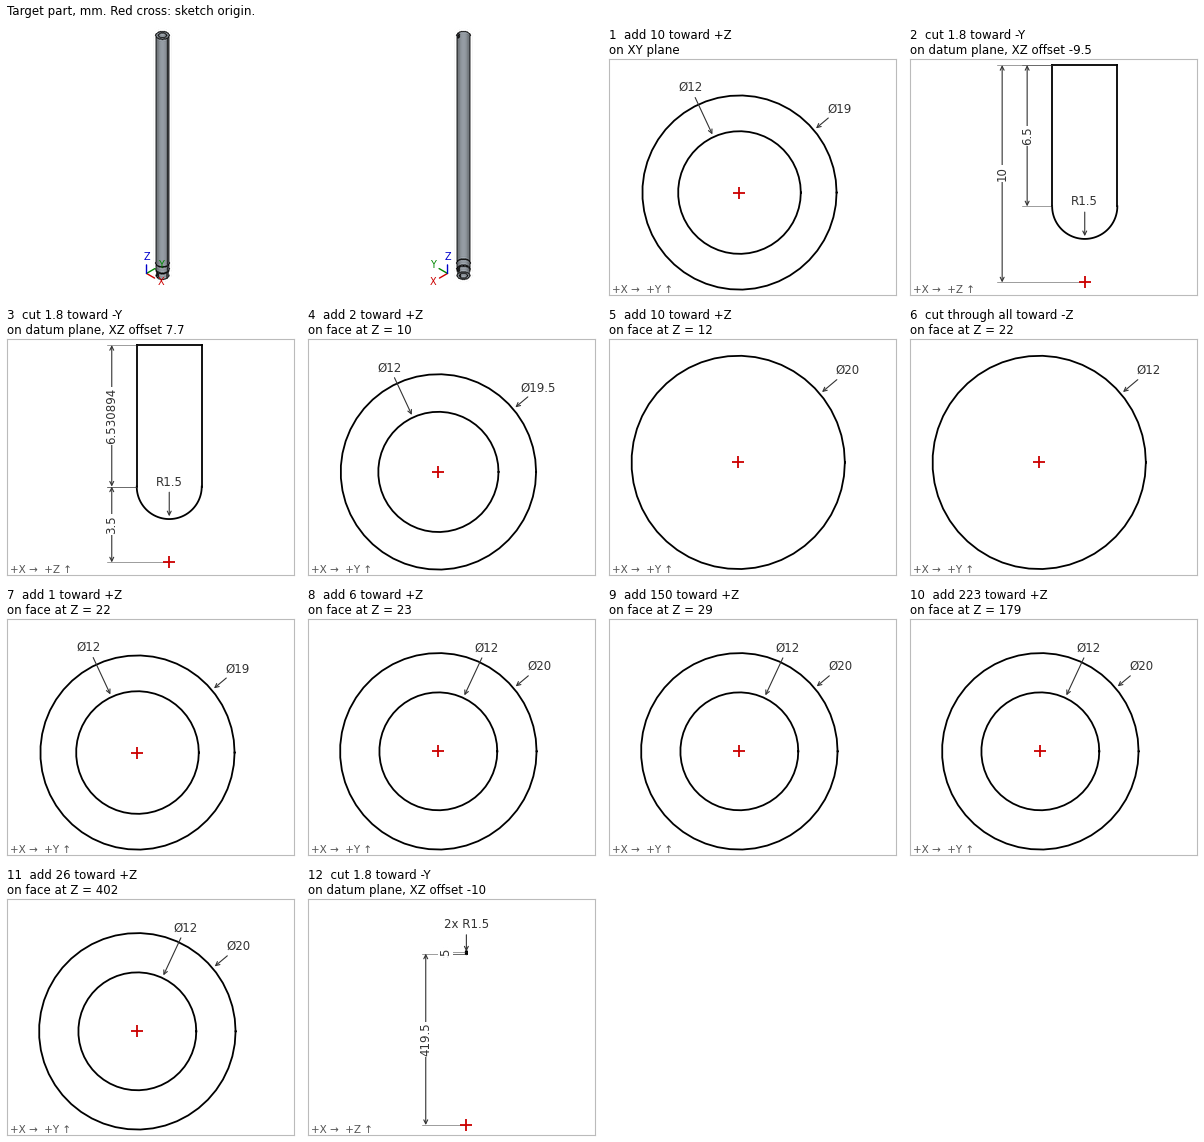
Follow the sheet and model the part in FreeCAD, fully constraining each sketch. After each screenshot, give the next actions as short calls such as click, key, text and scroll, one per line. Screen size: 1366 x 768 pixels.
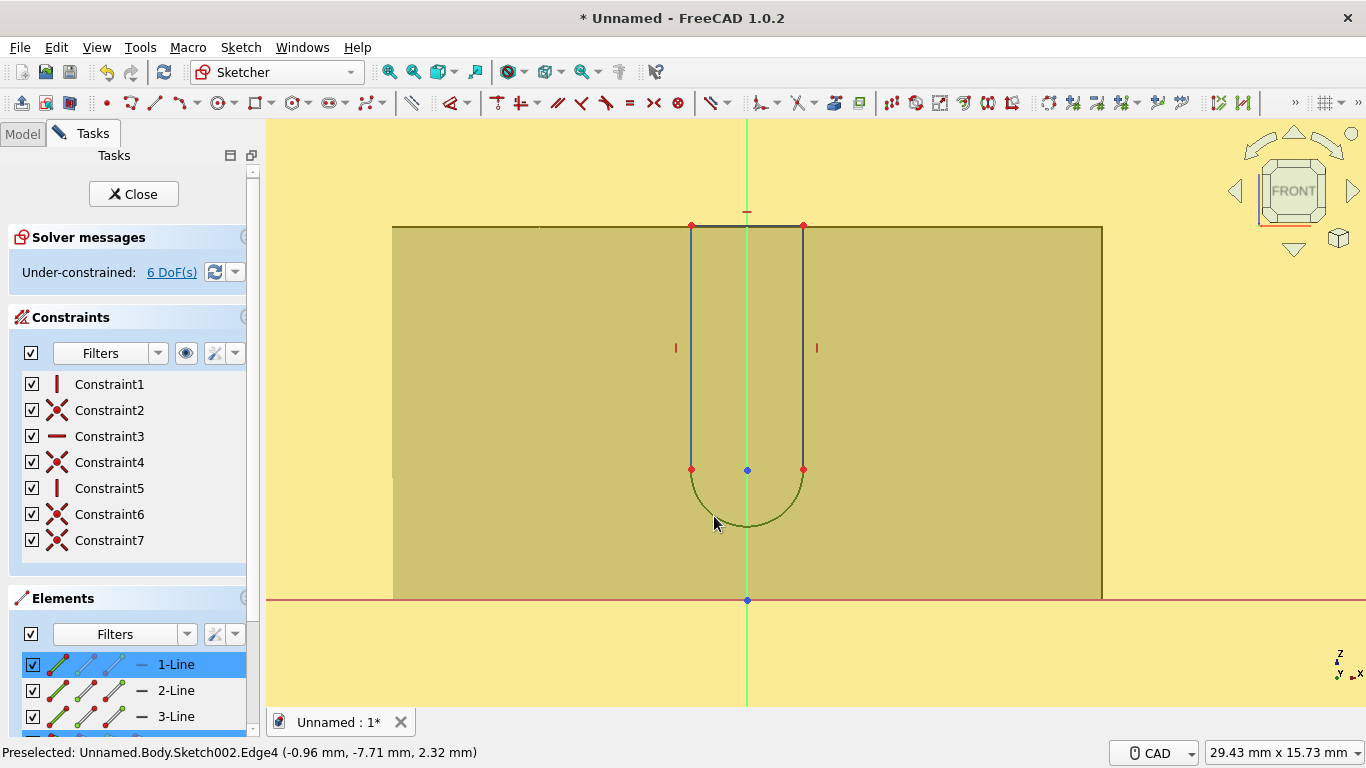
click(606, 104)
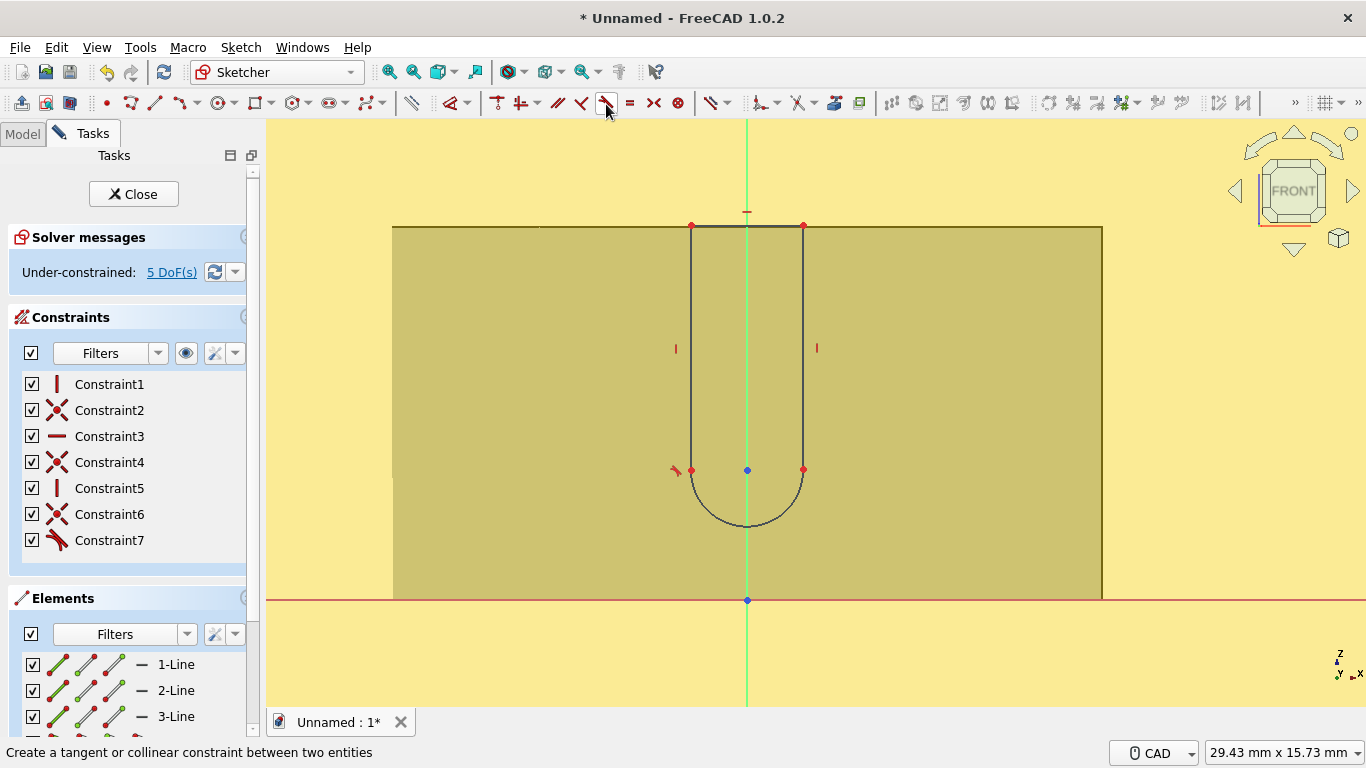
click(803, 299)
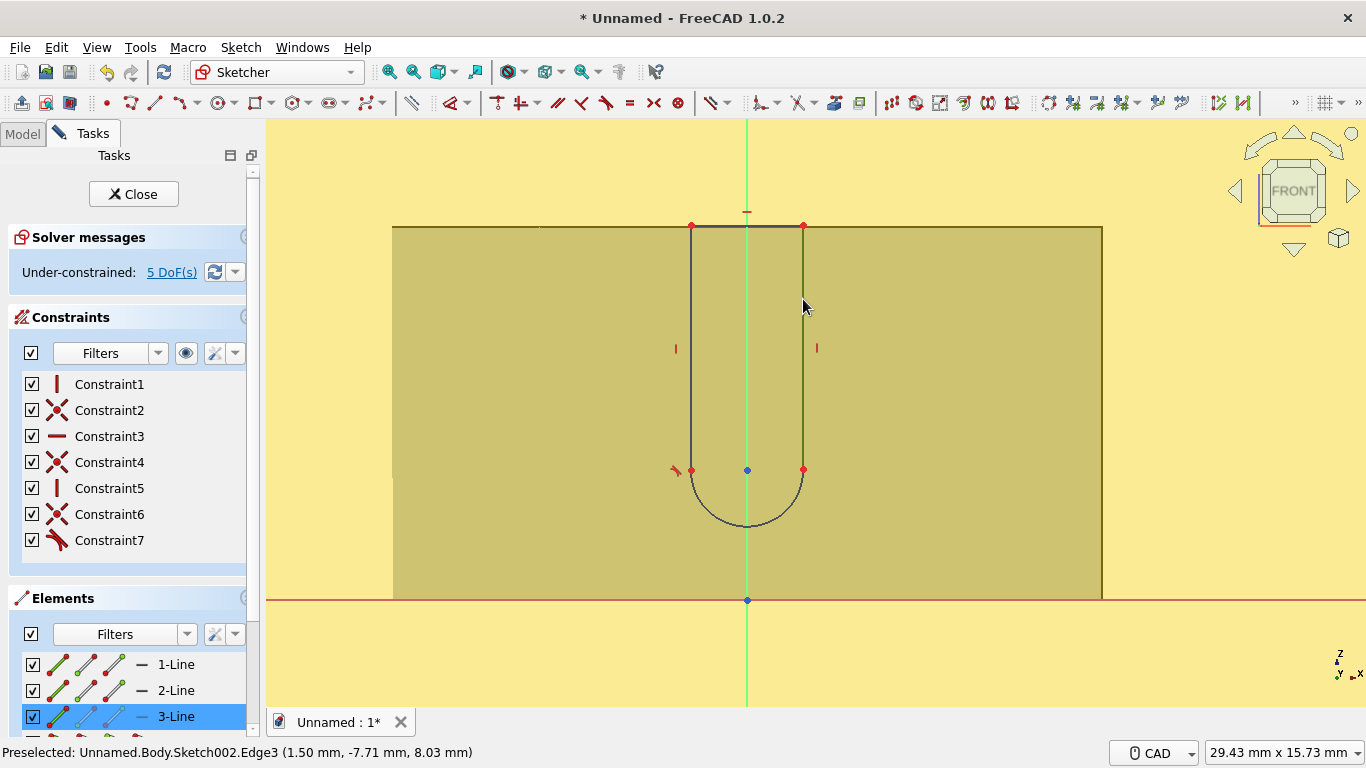
click(714, 516)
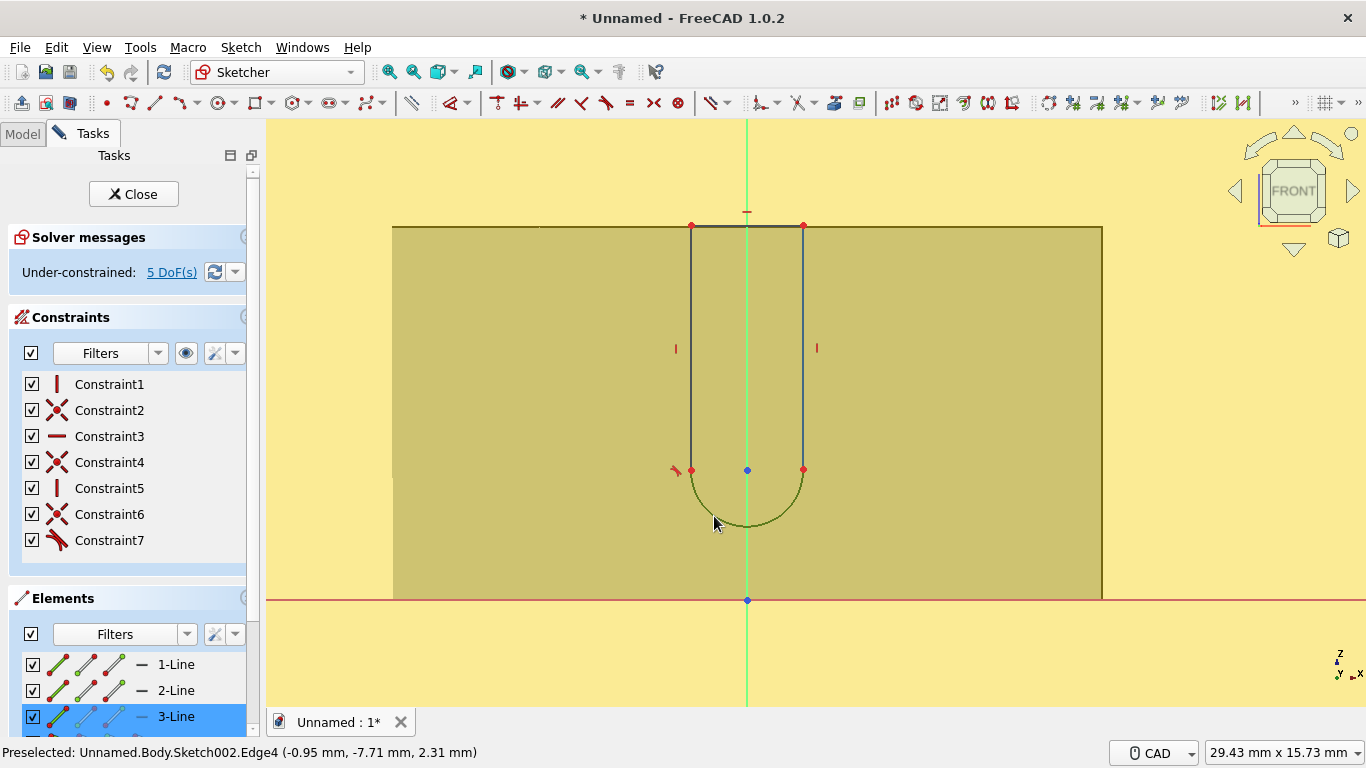
click(606, 104)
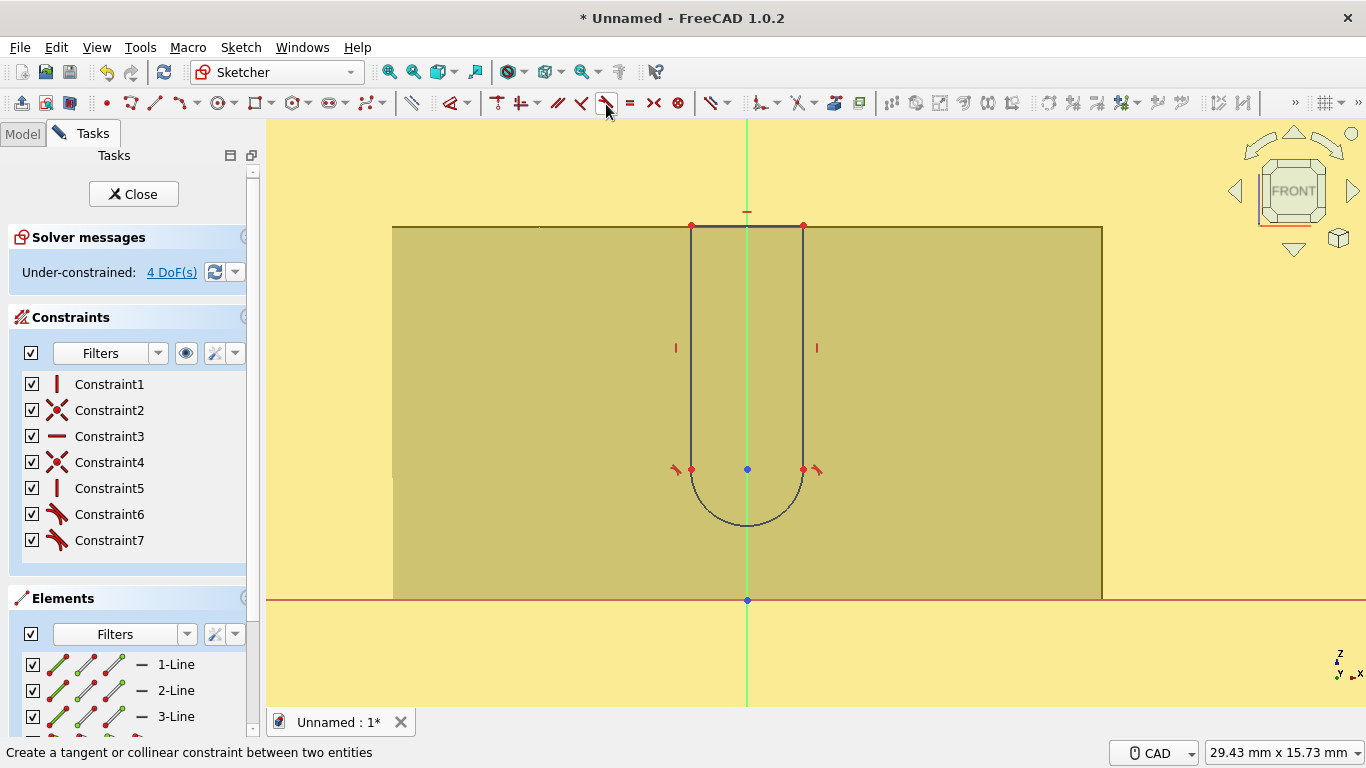
click(747, 470)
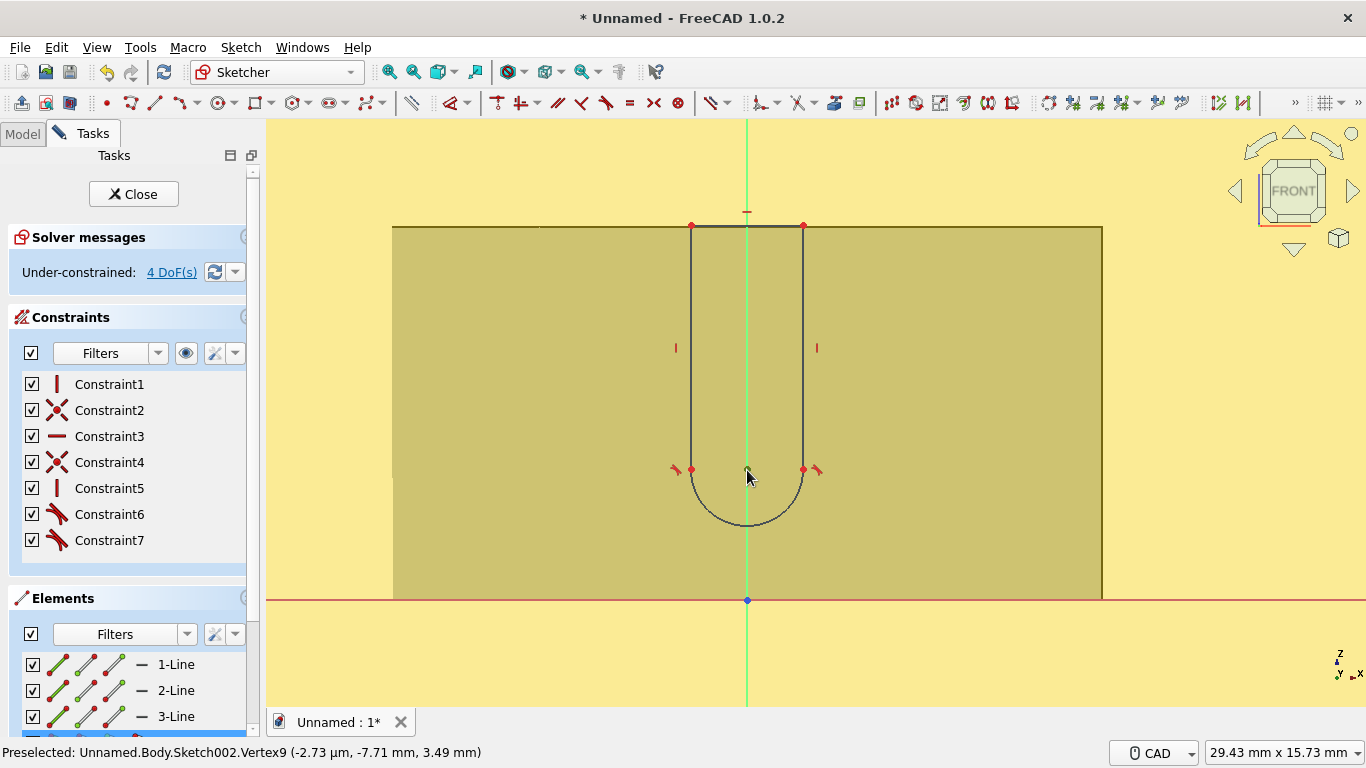
click(747, 641)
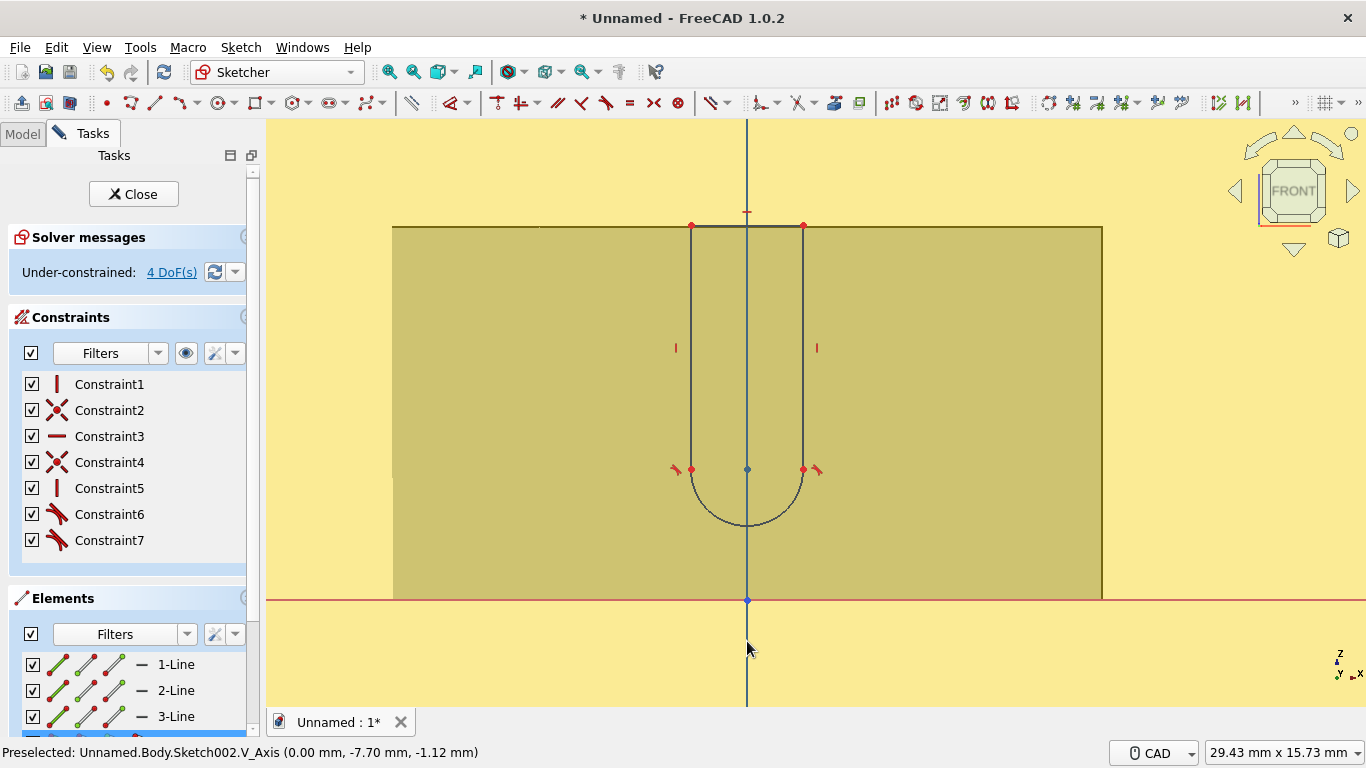
click(498, 104)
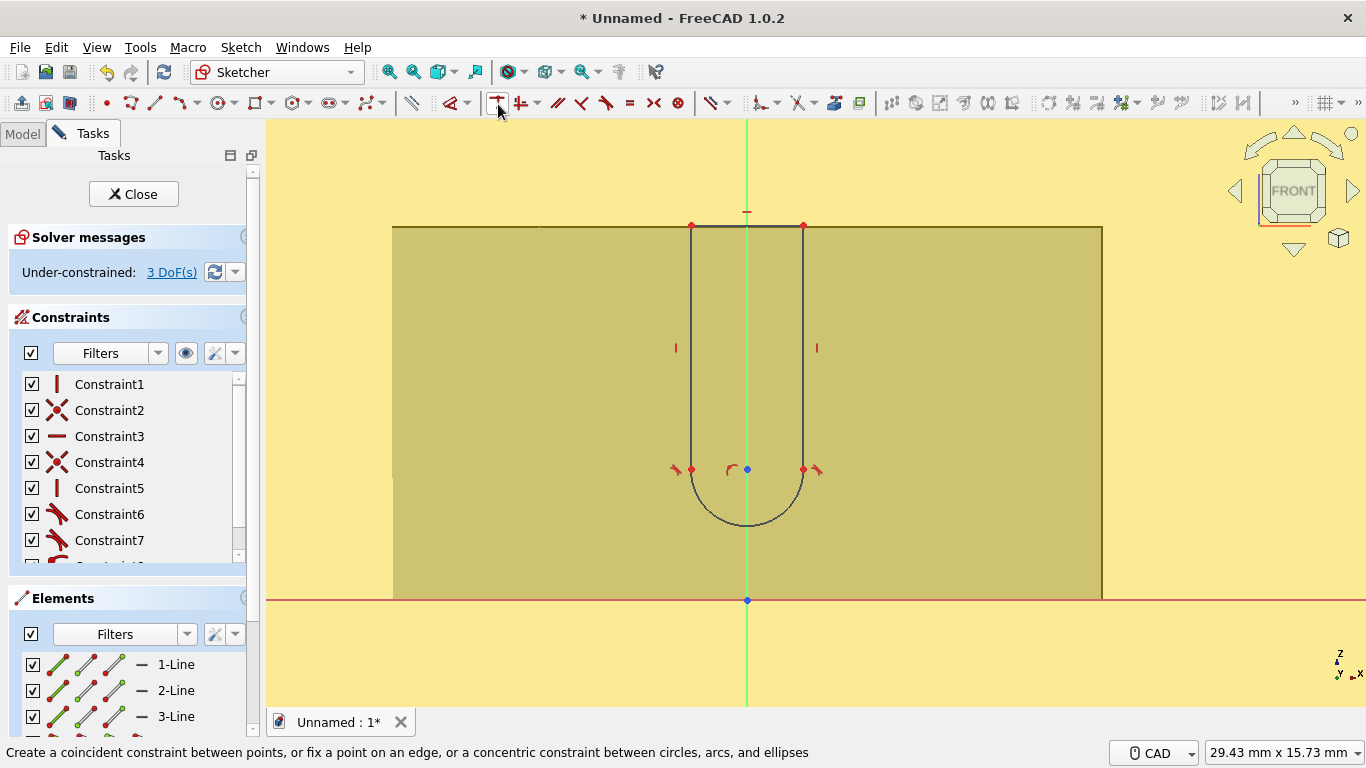
click(450, 104)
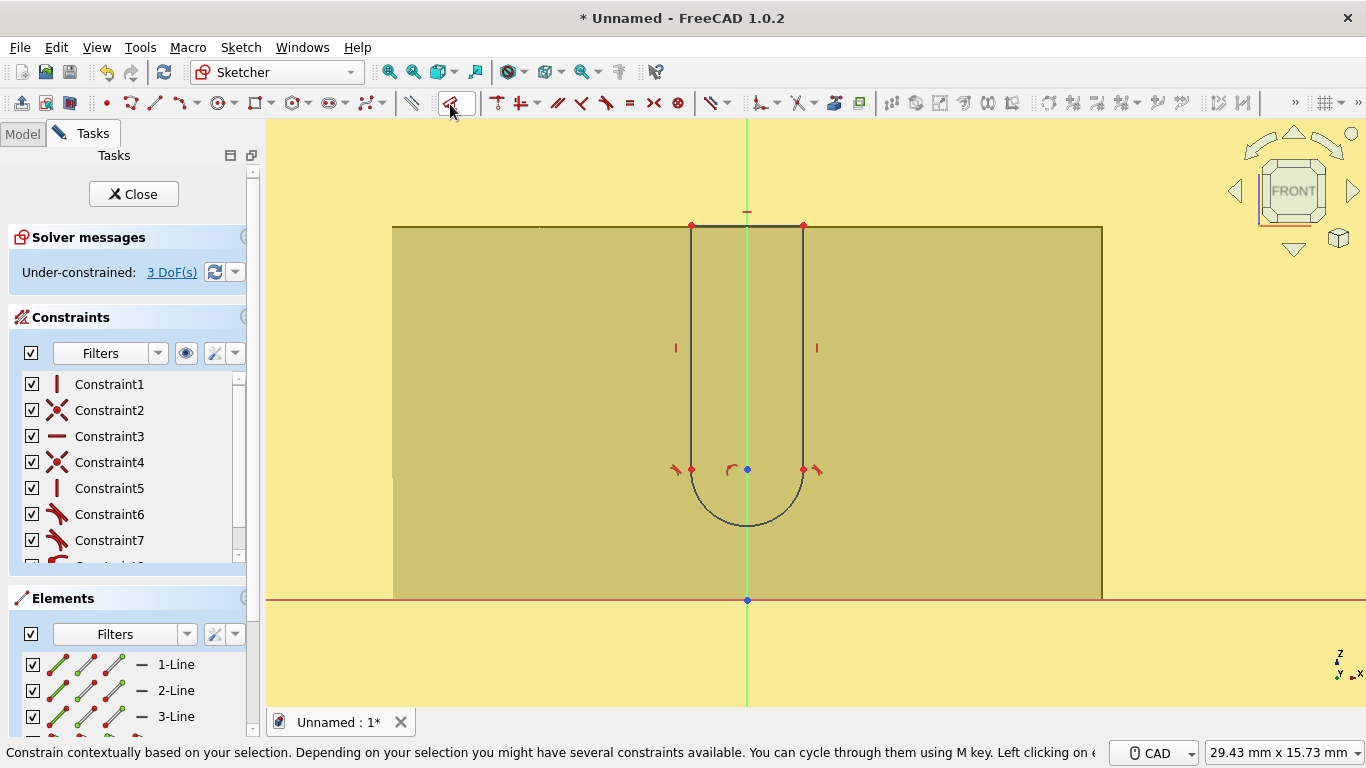
click(714, 515)
click(695, 541)